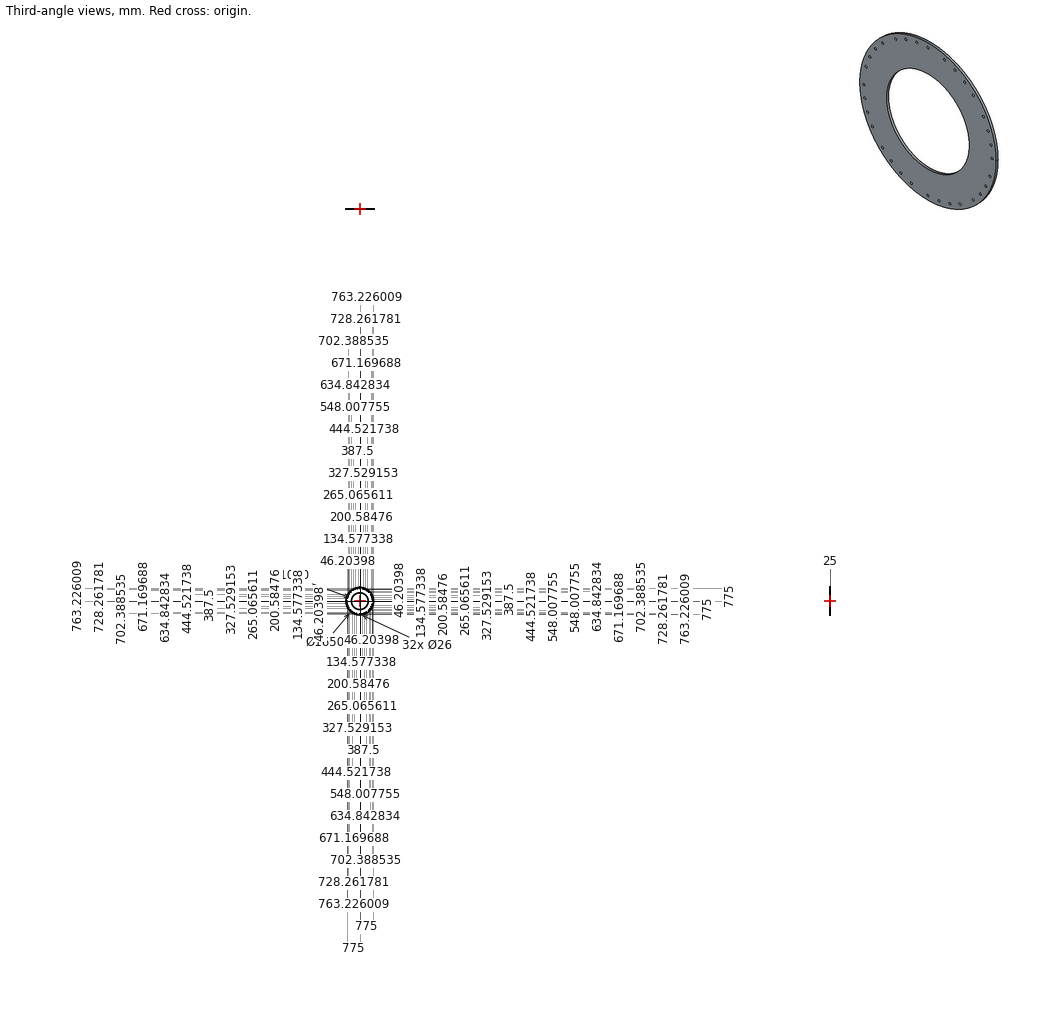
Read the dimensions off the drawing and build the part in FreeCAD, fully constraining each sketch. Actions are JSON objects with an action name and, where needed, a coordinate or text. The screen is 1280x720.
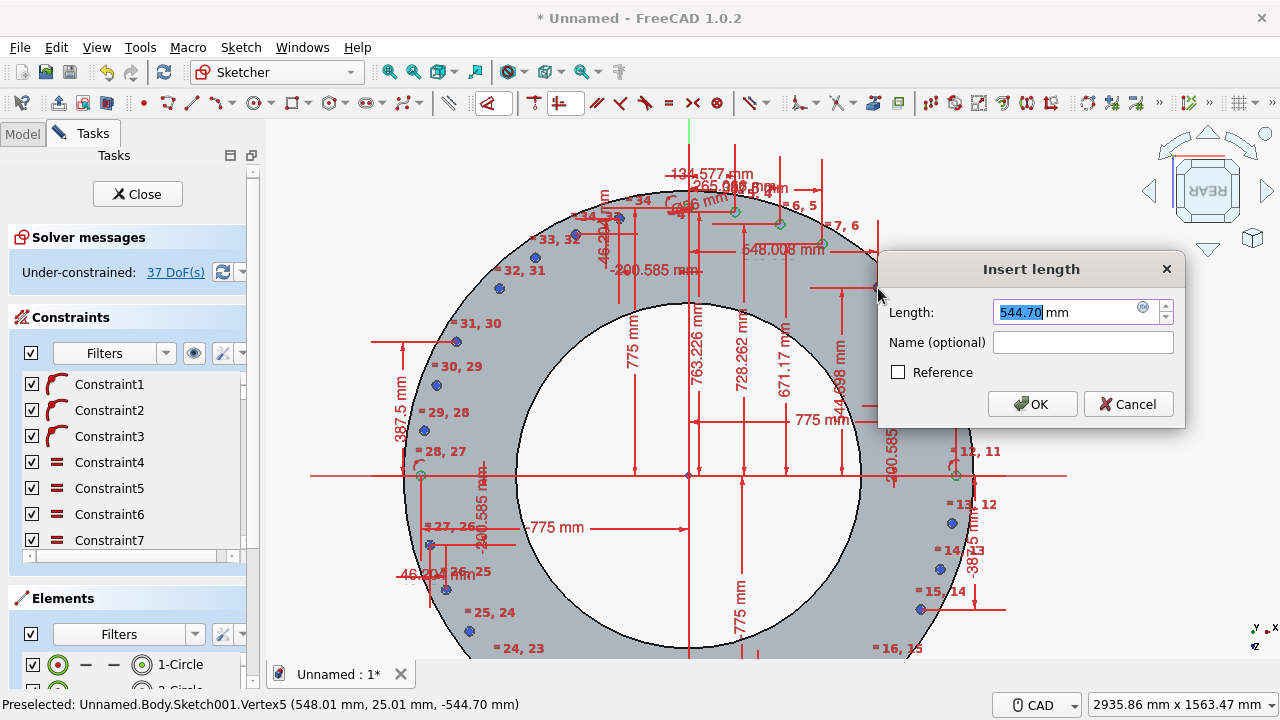
{"action": "type", "text": "548.007755"}
{"action": "key", "text": "Return"}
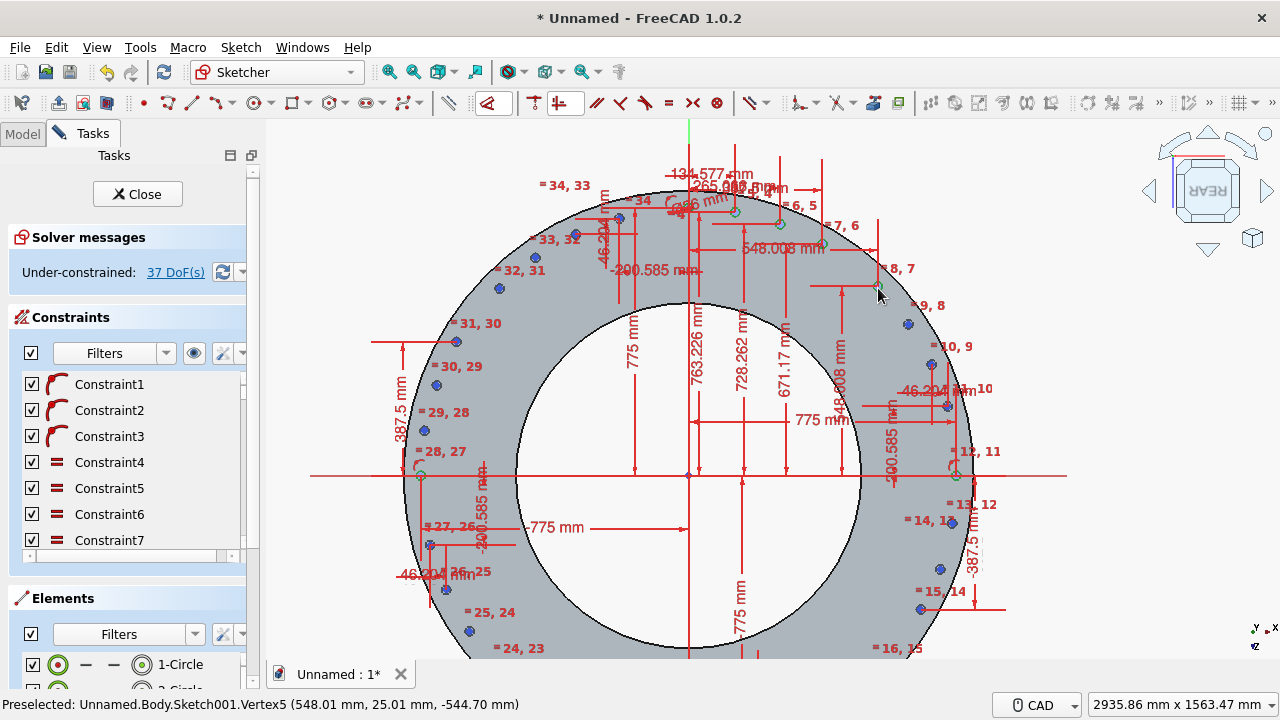
{"action": "left_click", "coordinate": [908, 324]}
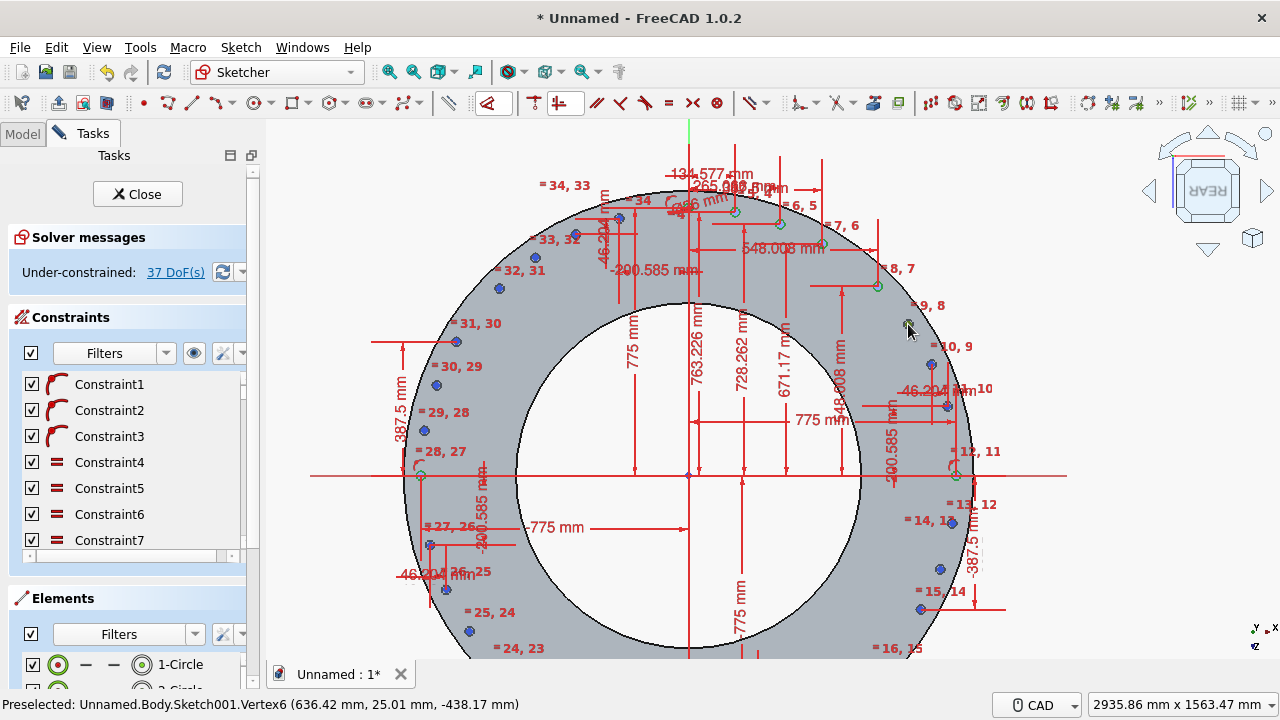
{"action": "key", "text": "l"}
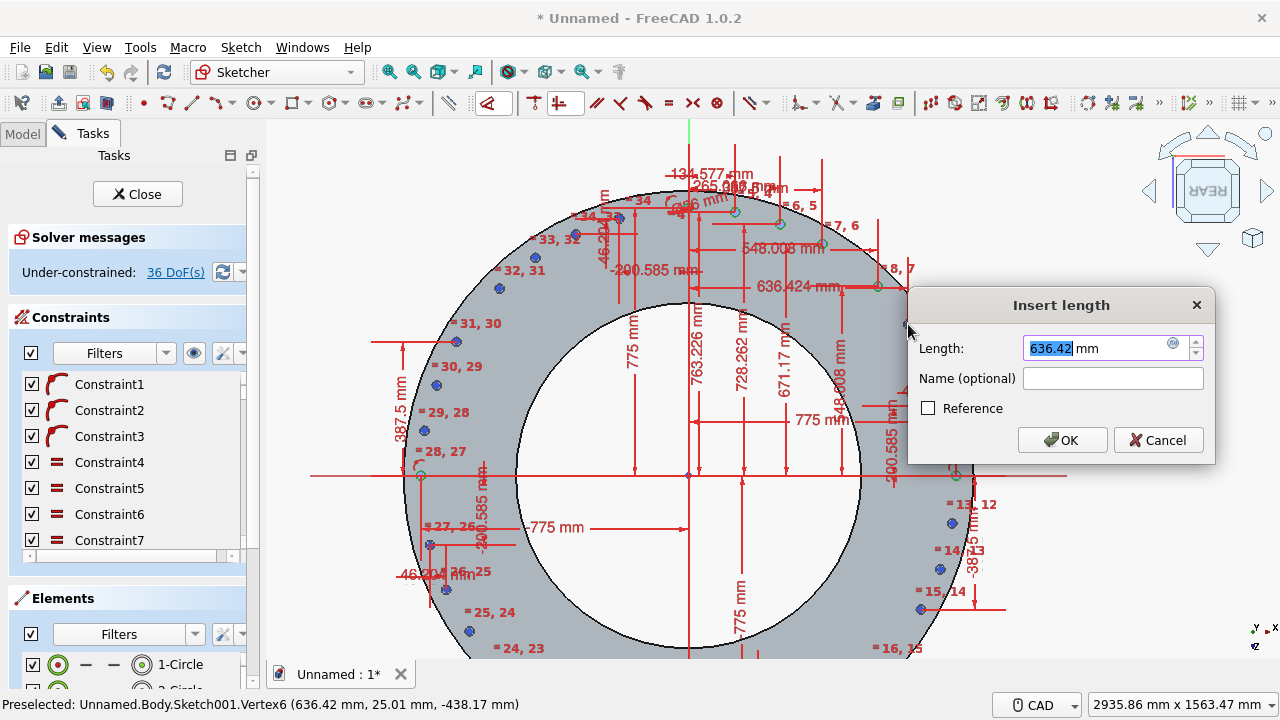
{"action": "type", "text": "634.842834"}
{"action": "key", "text": "Return"}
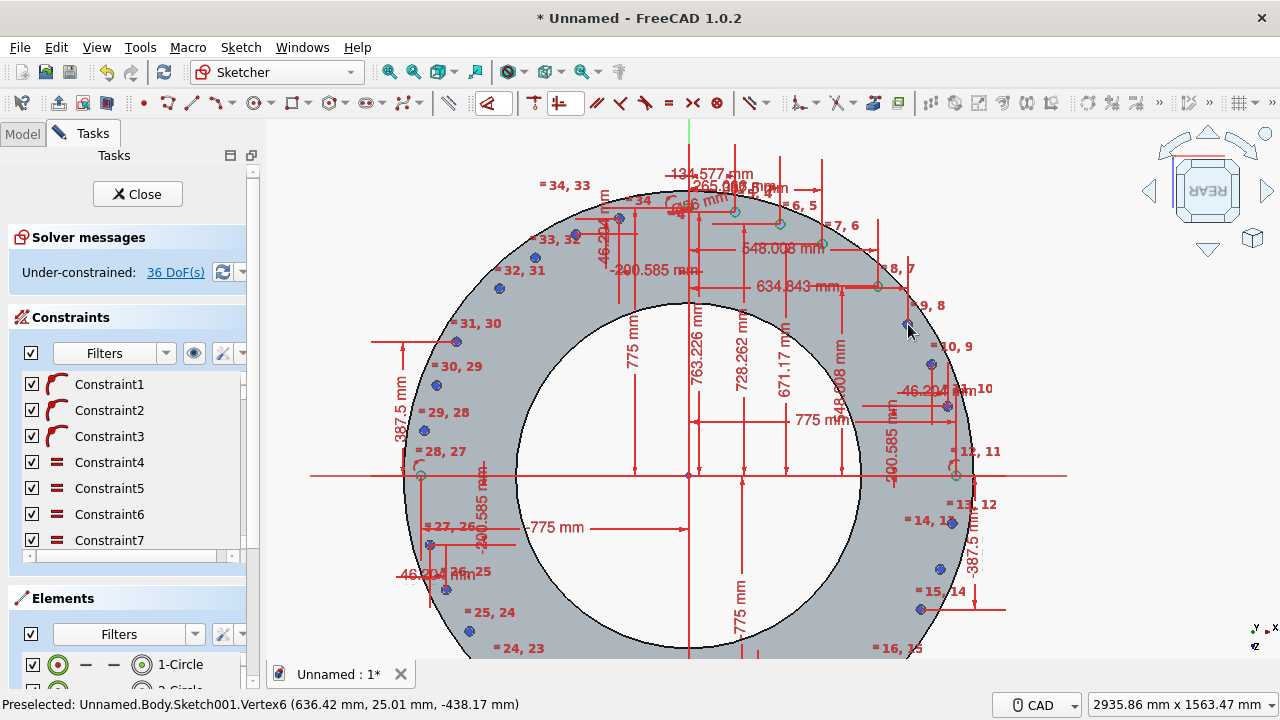
{"action": "left_click", "coordinate": [908, 324]}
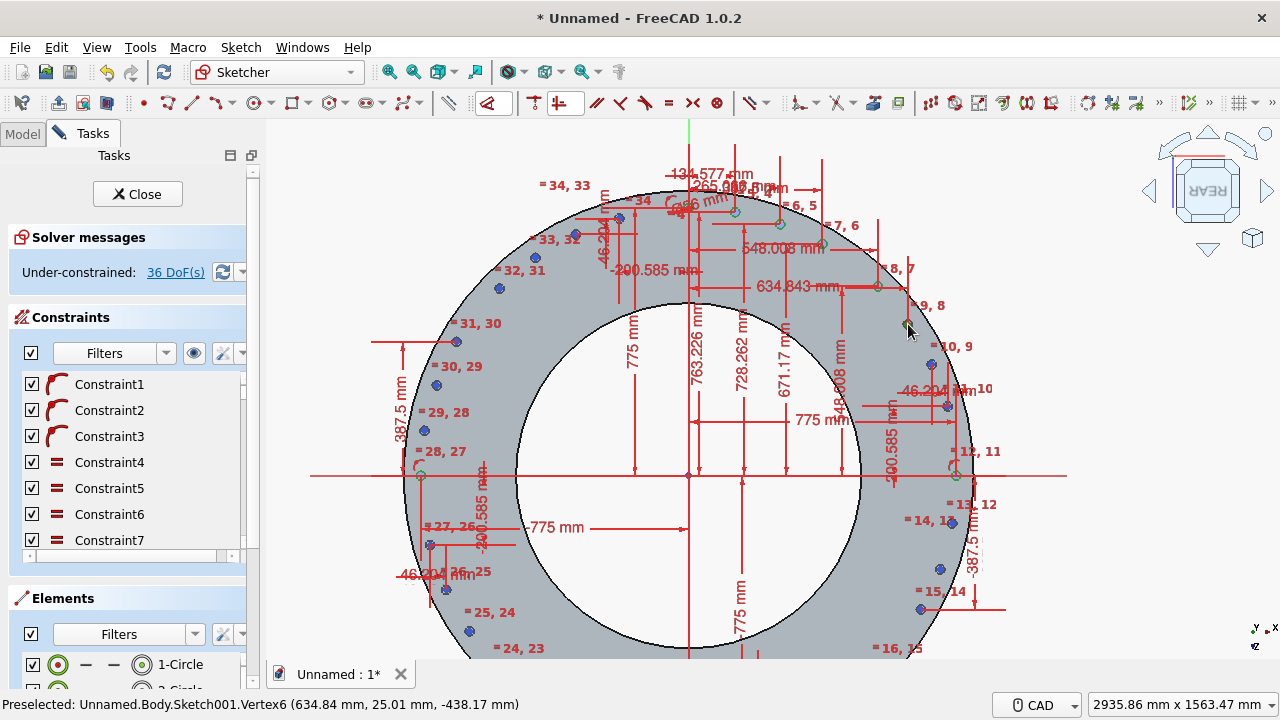
{"action": "key", "text": "i"}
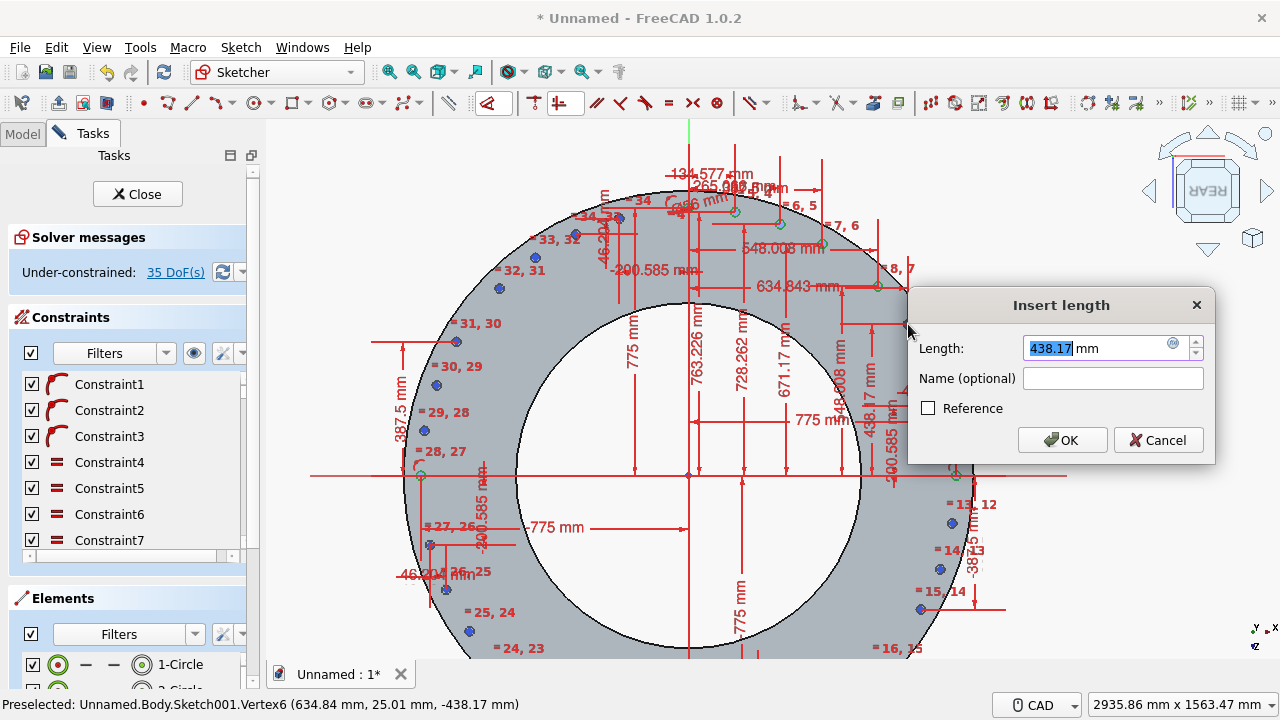
{"action": "type", "text": "444.521738"}
{"action": "key", "text": "Return"}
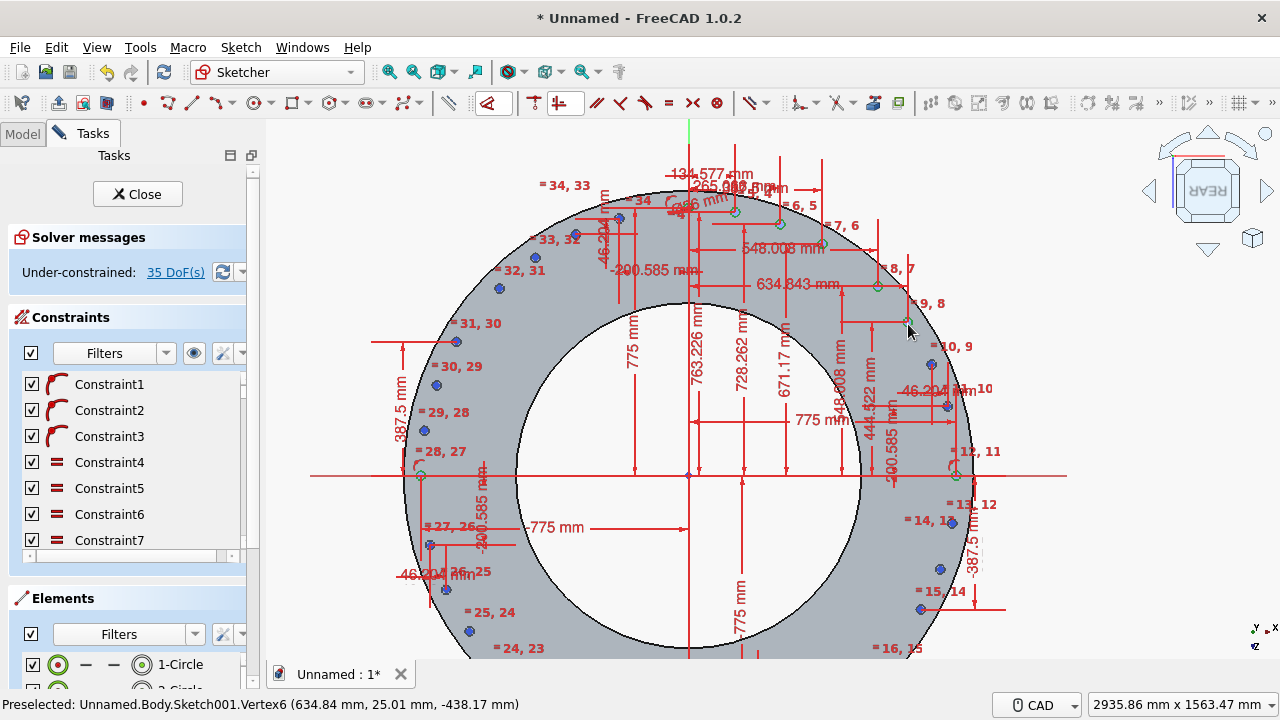
{"action": "left_click", "coordinate": [932, 365]}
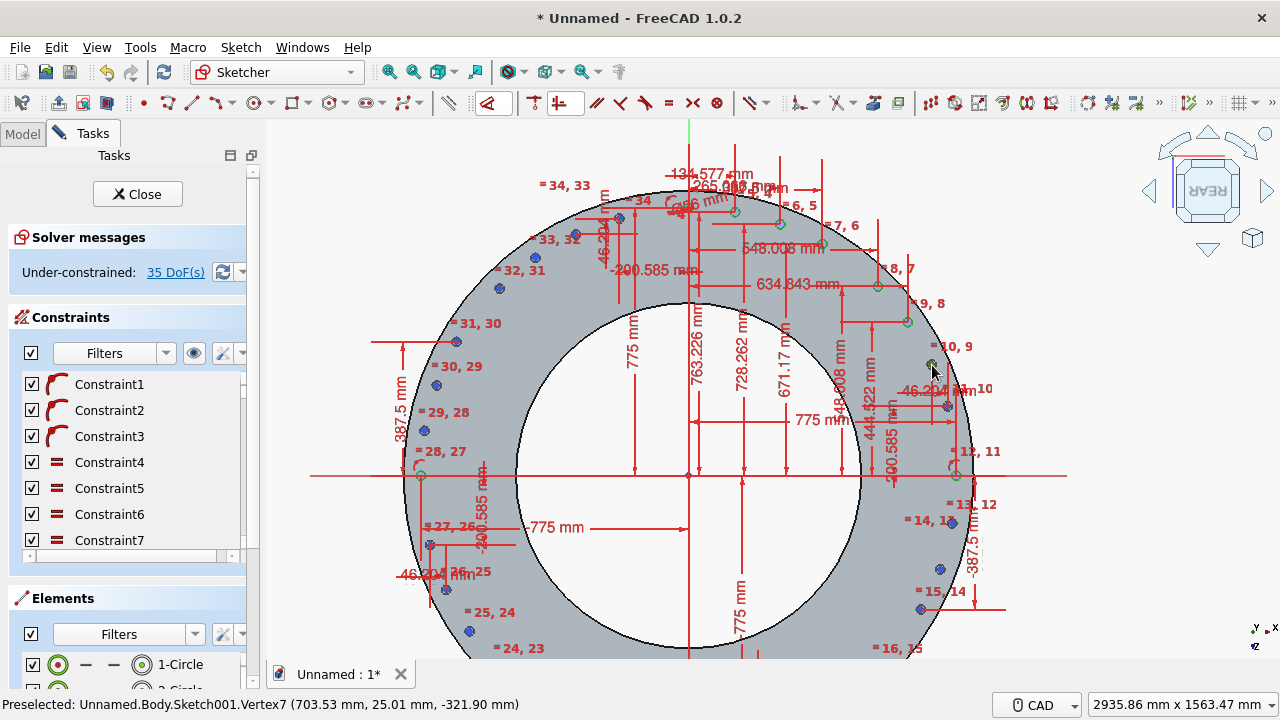
{"action": "key", "text": "l"}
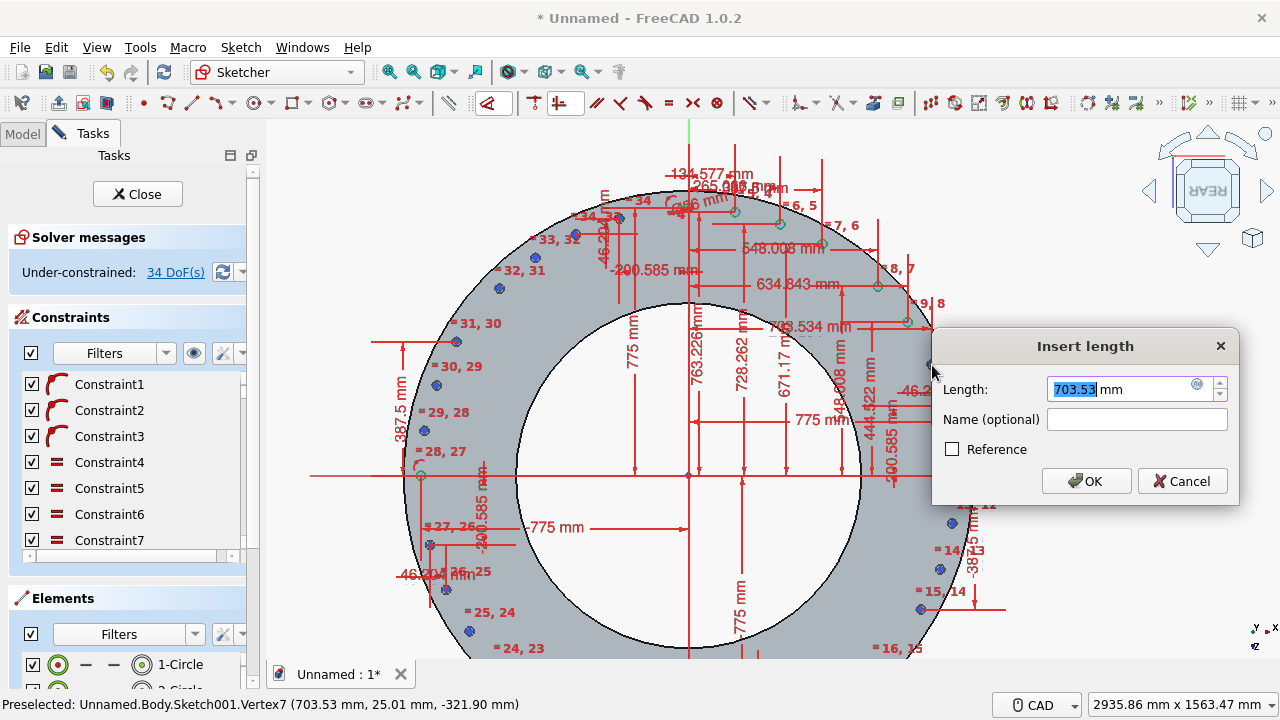
{"action": "type", "text": "702.388535"}
{"action": "key", "text": "Return"}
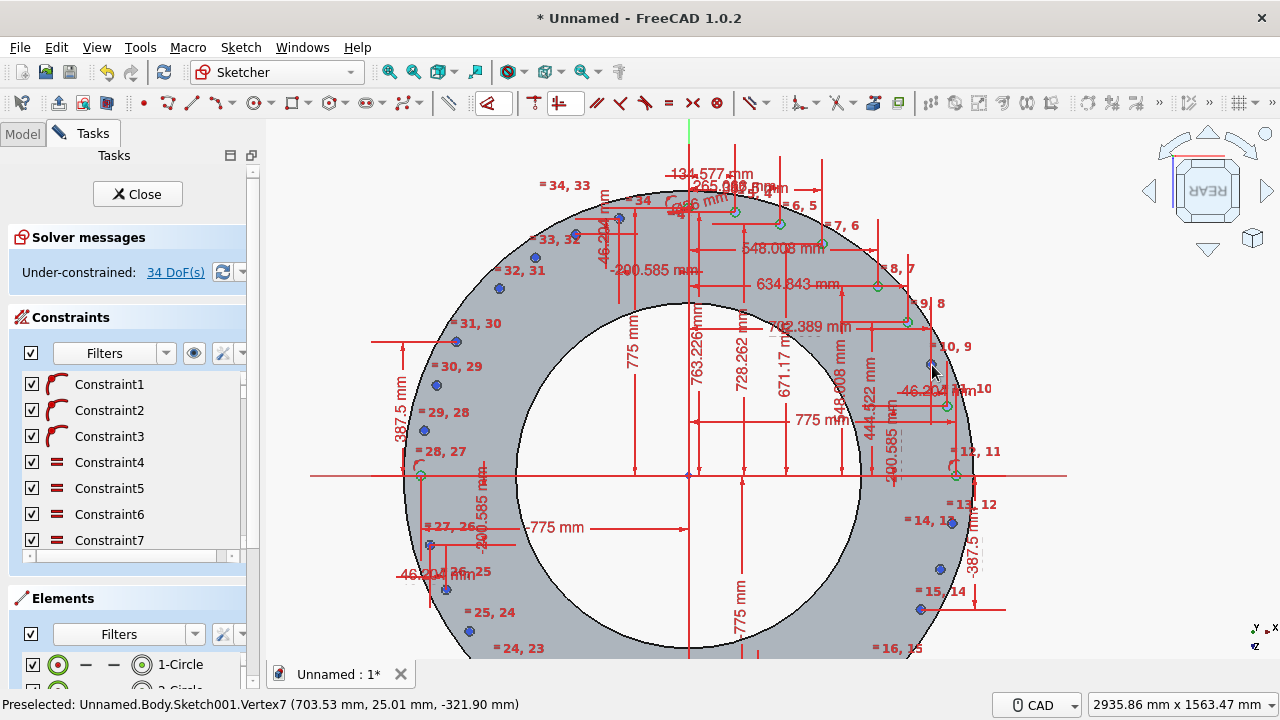
{"action": "left_click", "coordinate": [931, 365]}